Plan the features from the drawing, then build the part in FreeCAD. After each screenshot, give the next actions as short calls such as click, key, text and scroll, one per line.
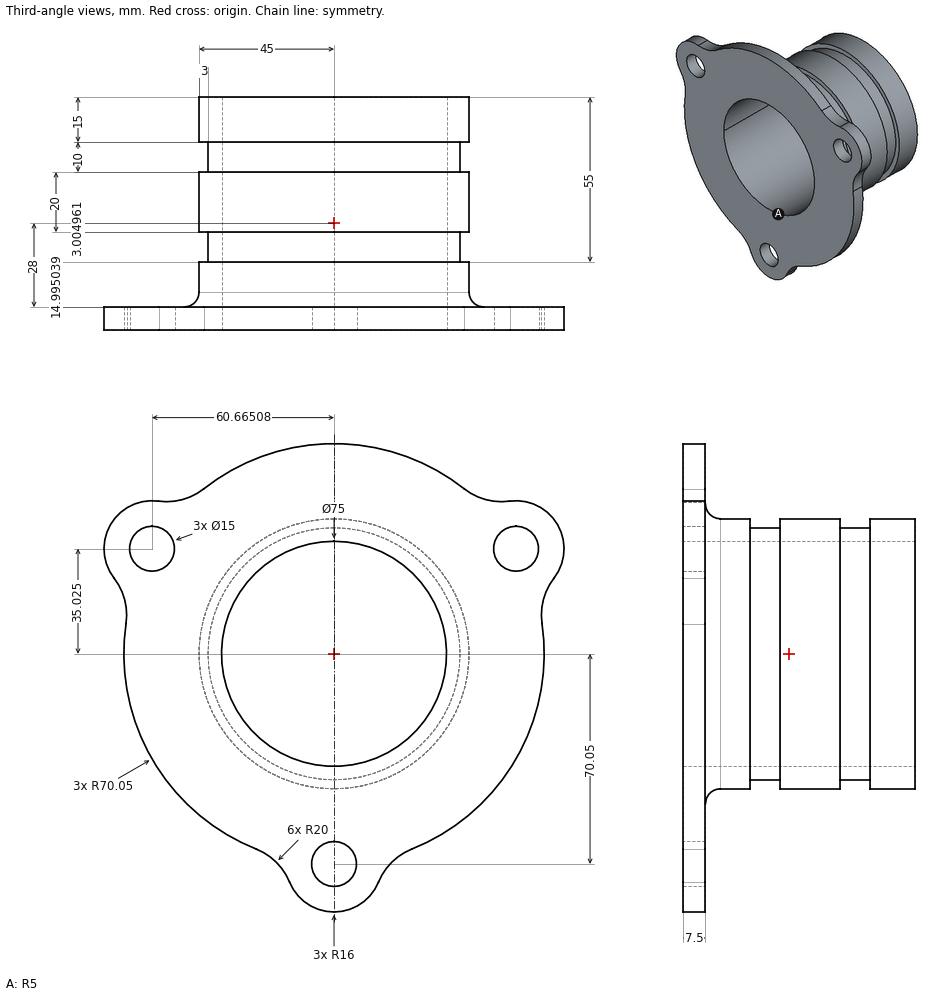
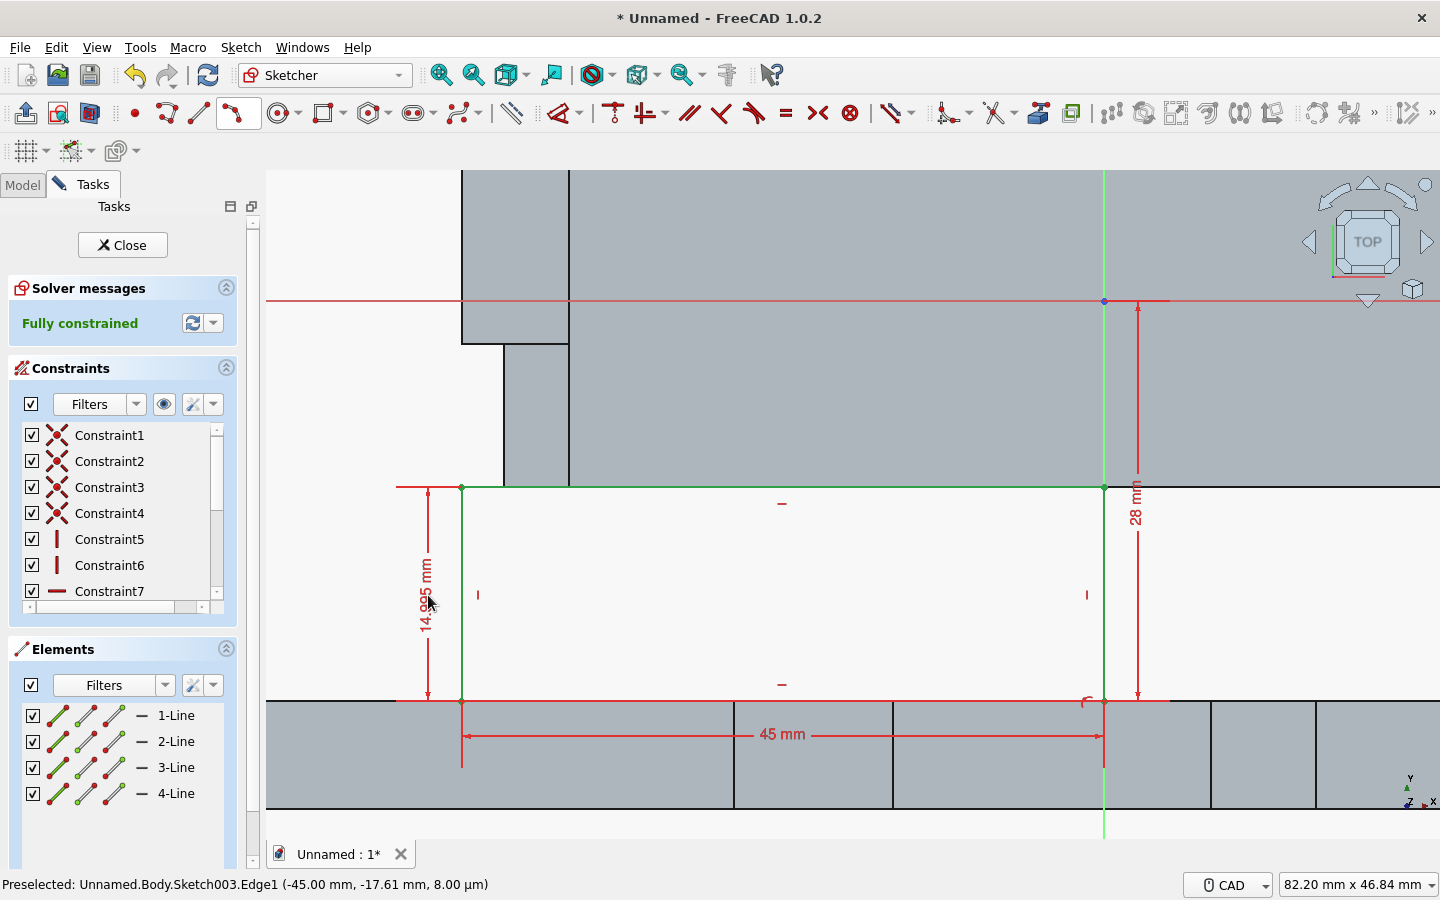
click(123, 245)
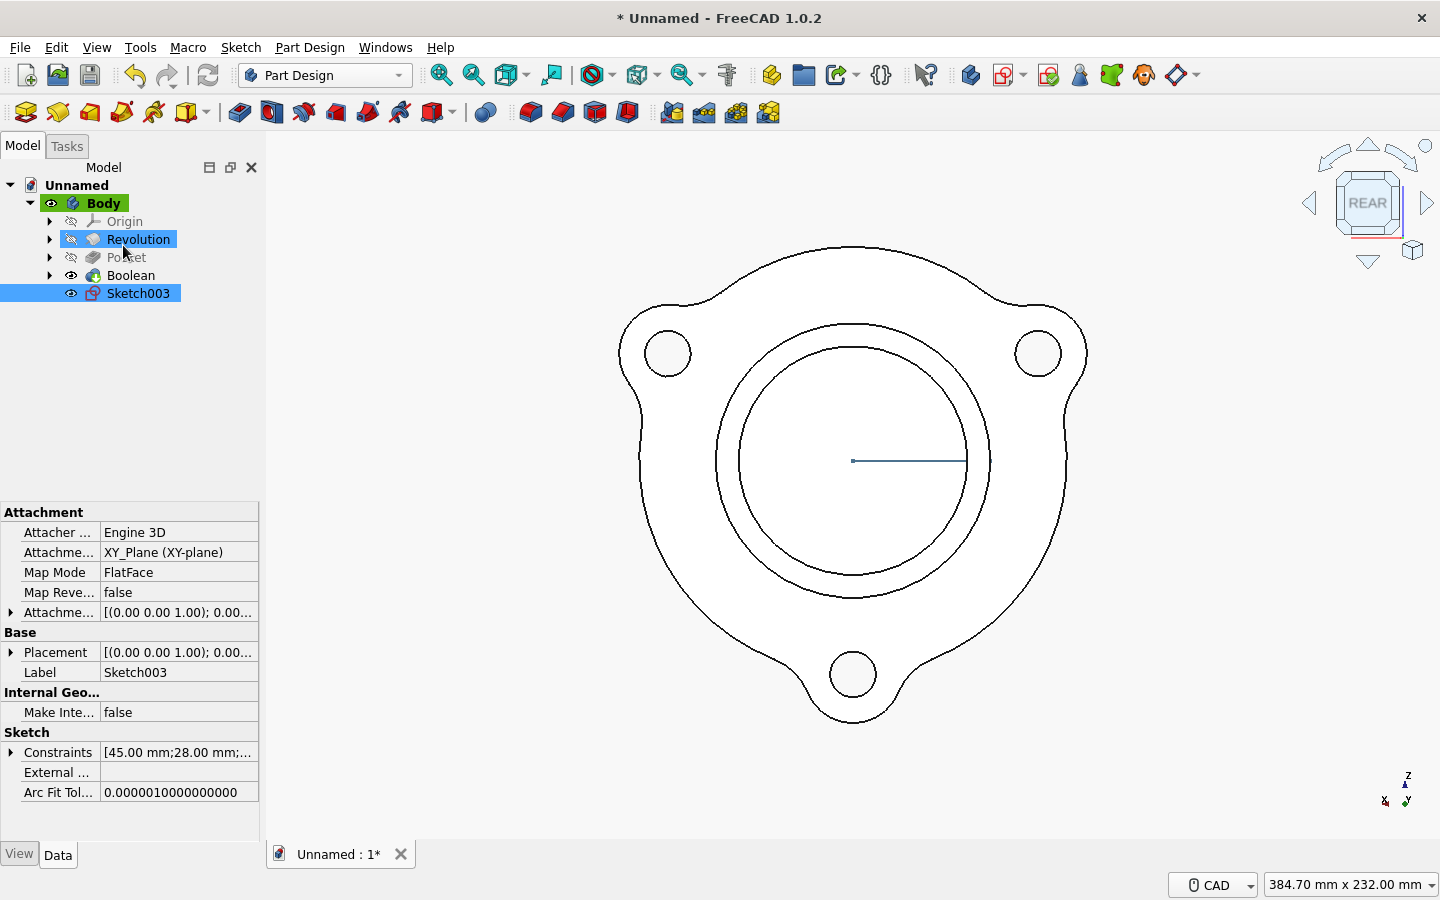
click(58, 112)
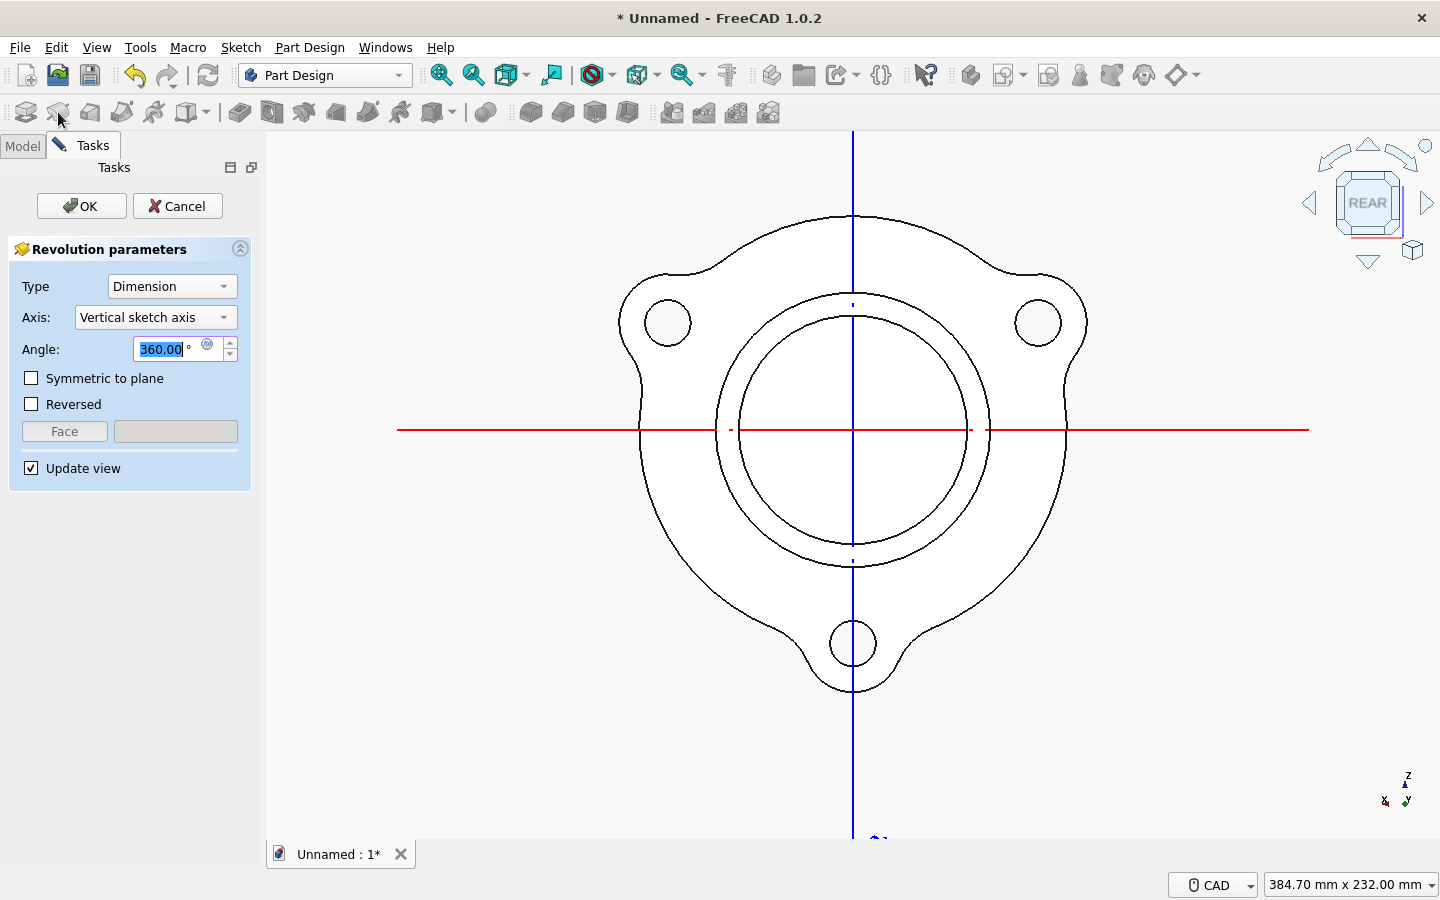
click(82, 206)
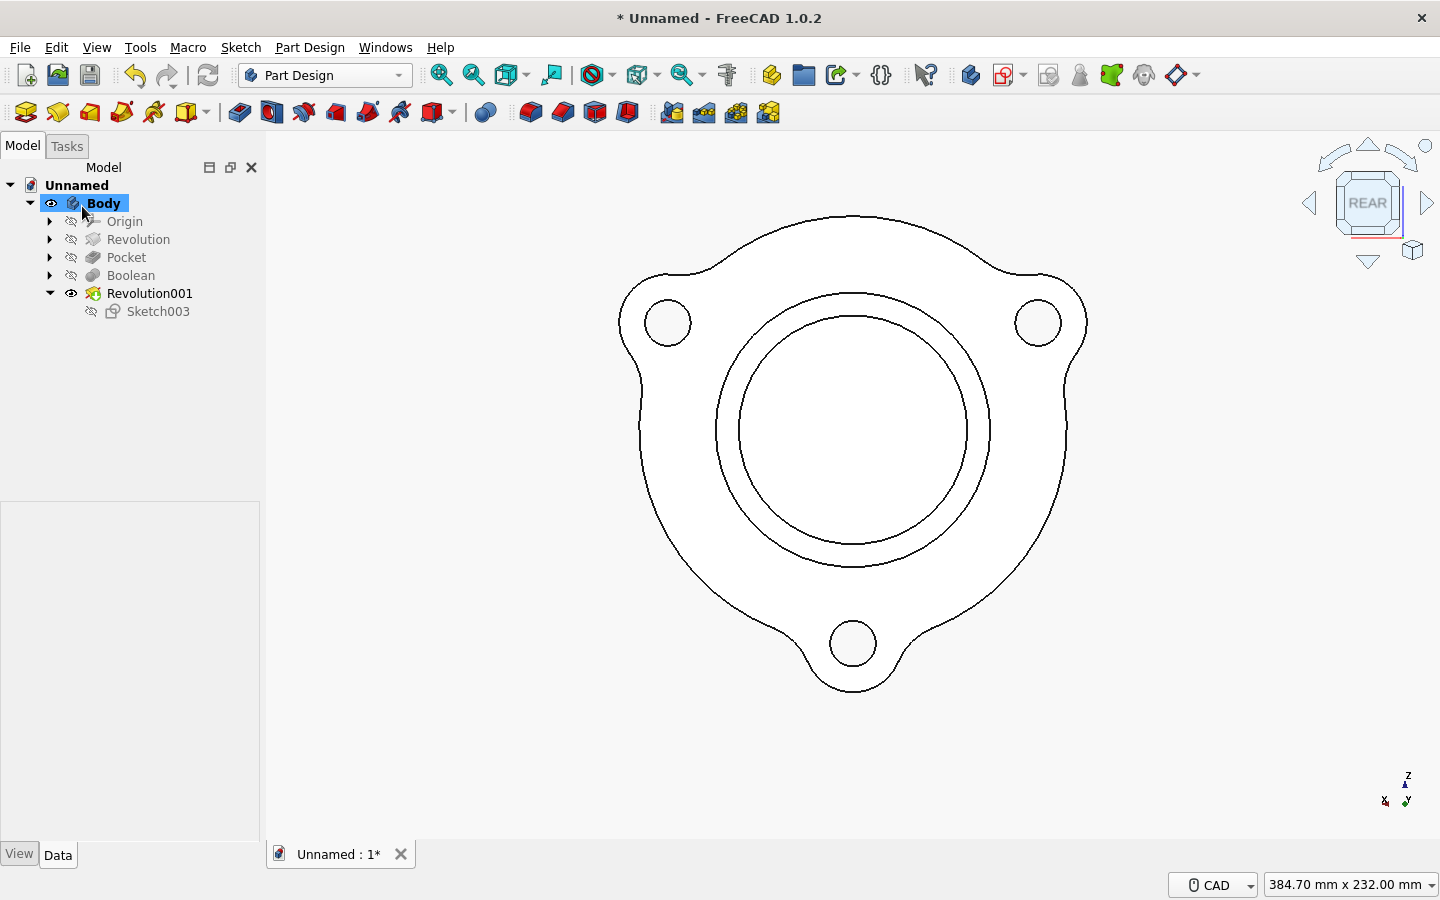
click(892, 547)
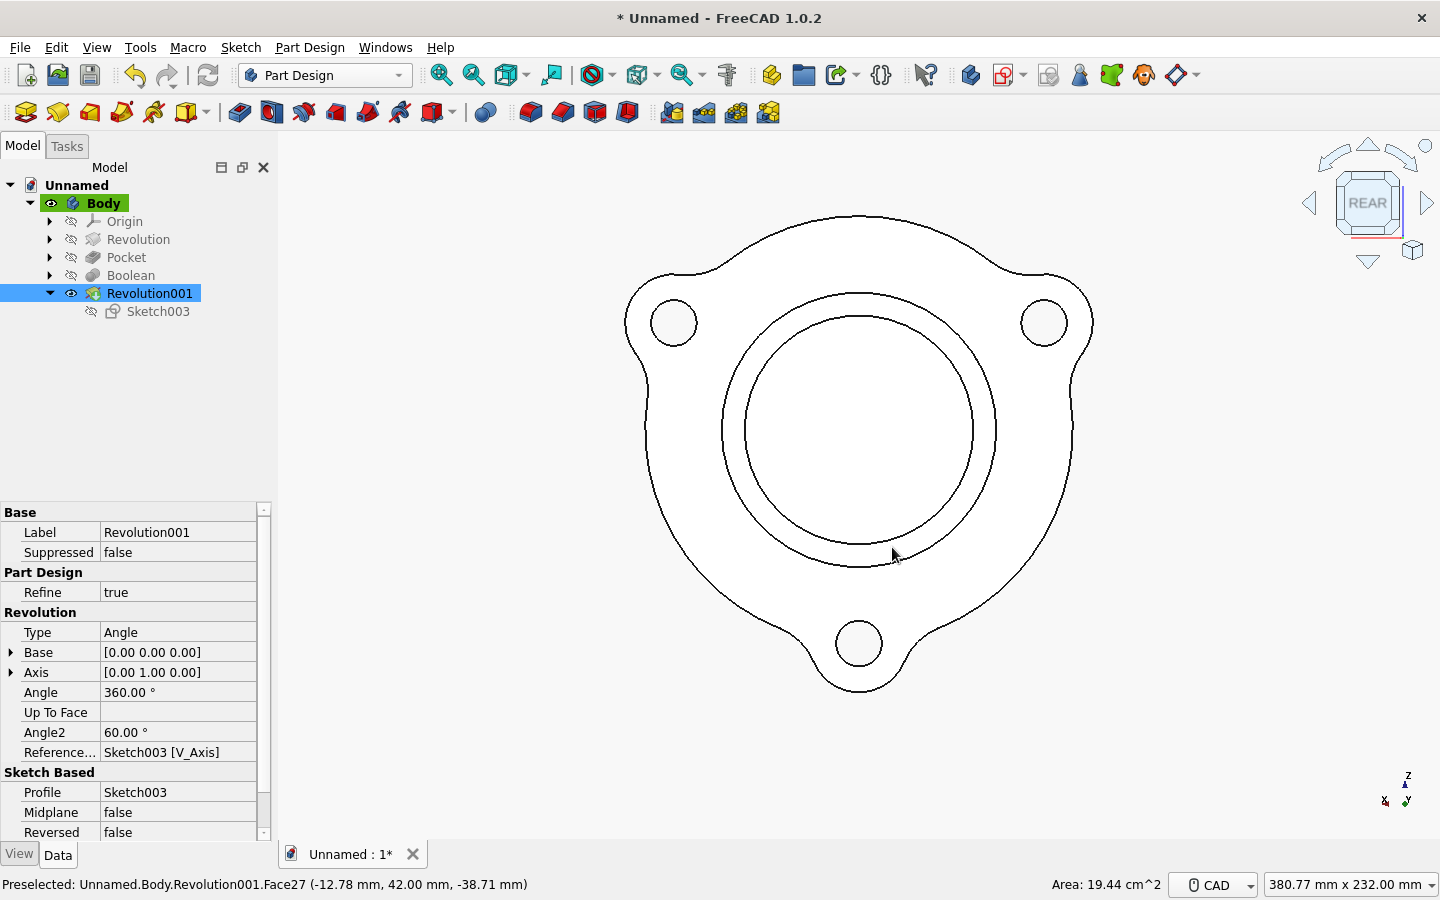
click(1004, 76)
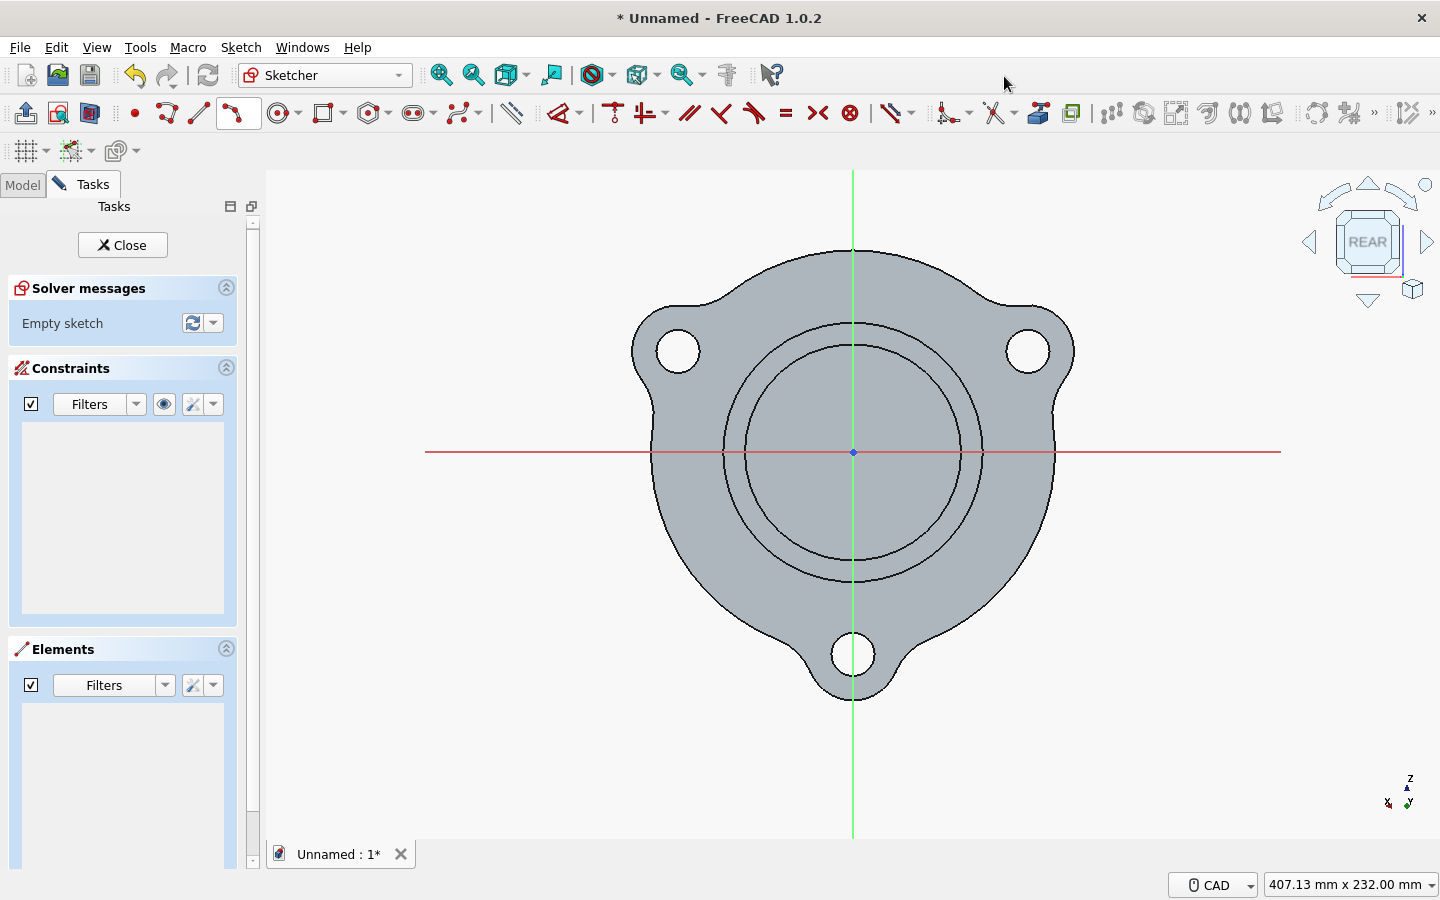
scroll(936, 389, up, 3)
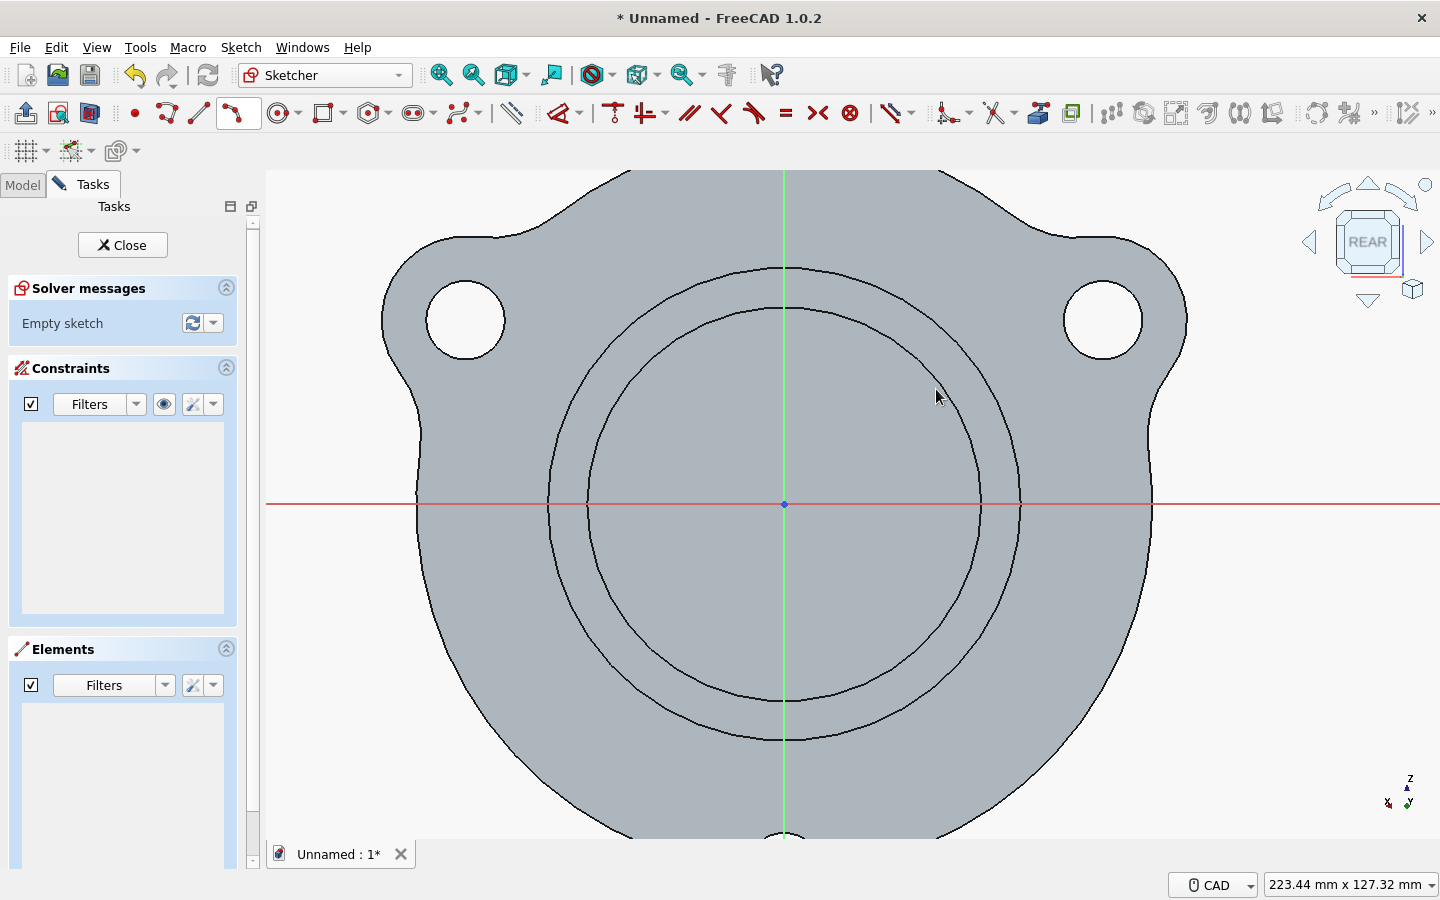
click(278, 114)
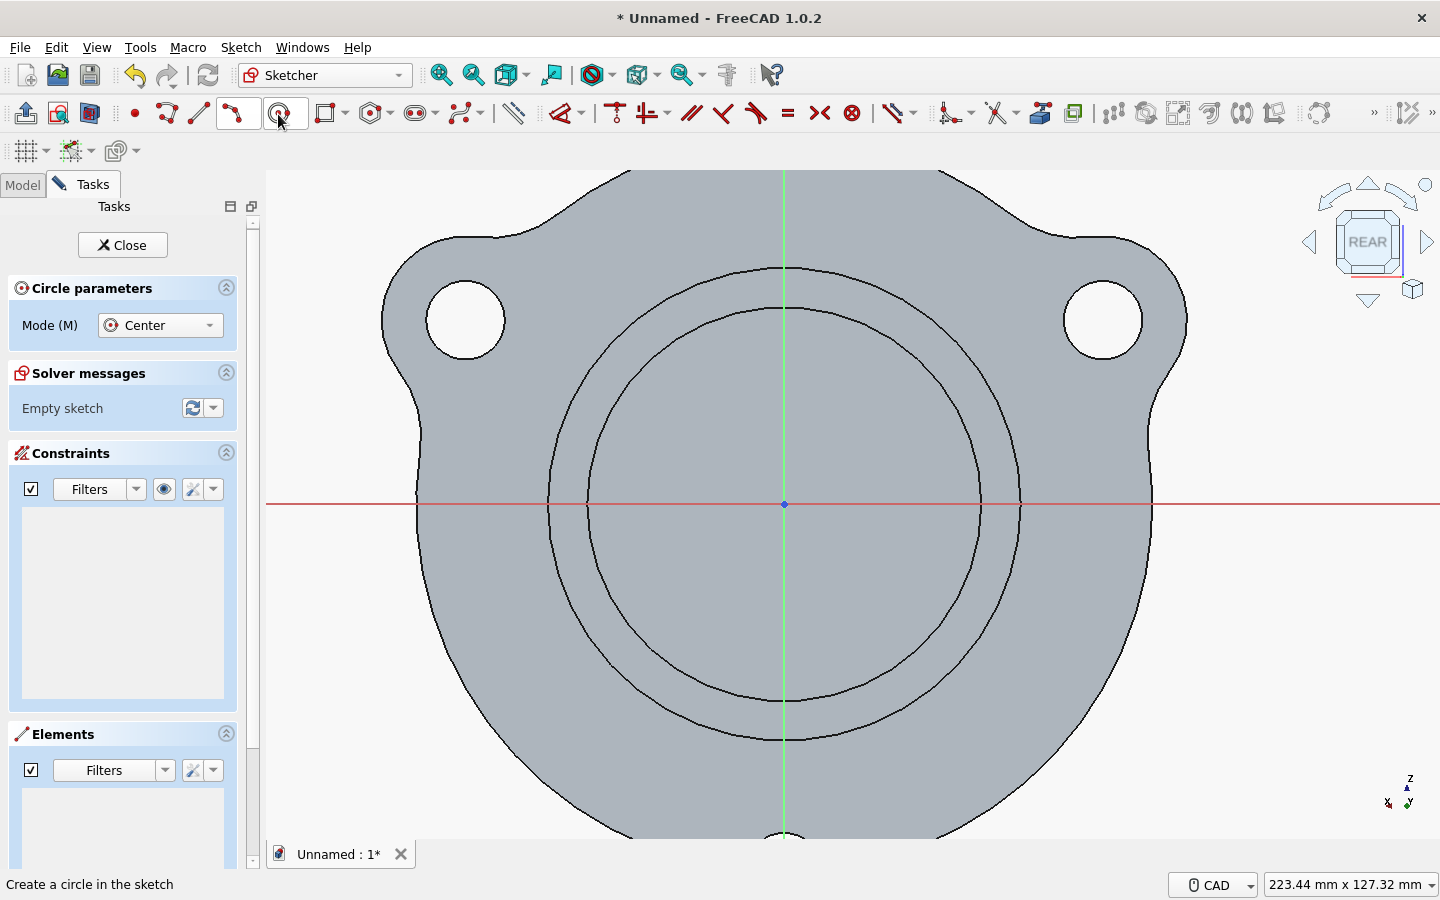
click(784, 504)
click(924, 365)
key(Escape)